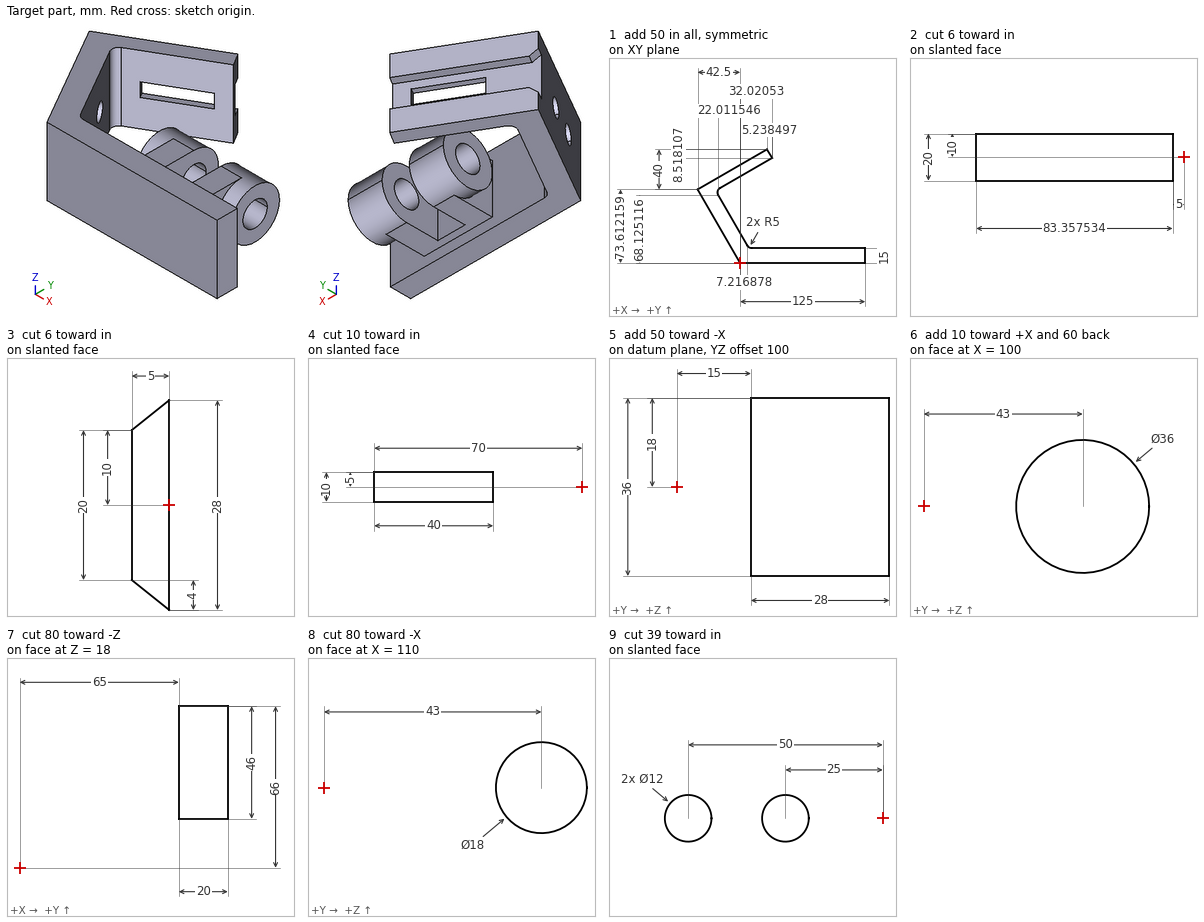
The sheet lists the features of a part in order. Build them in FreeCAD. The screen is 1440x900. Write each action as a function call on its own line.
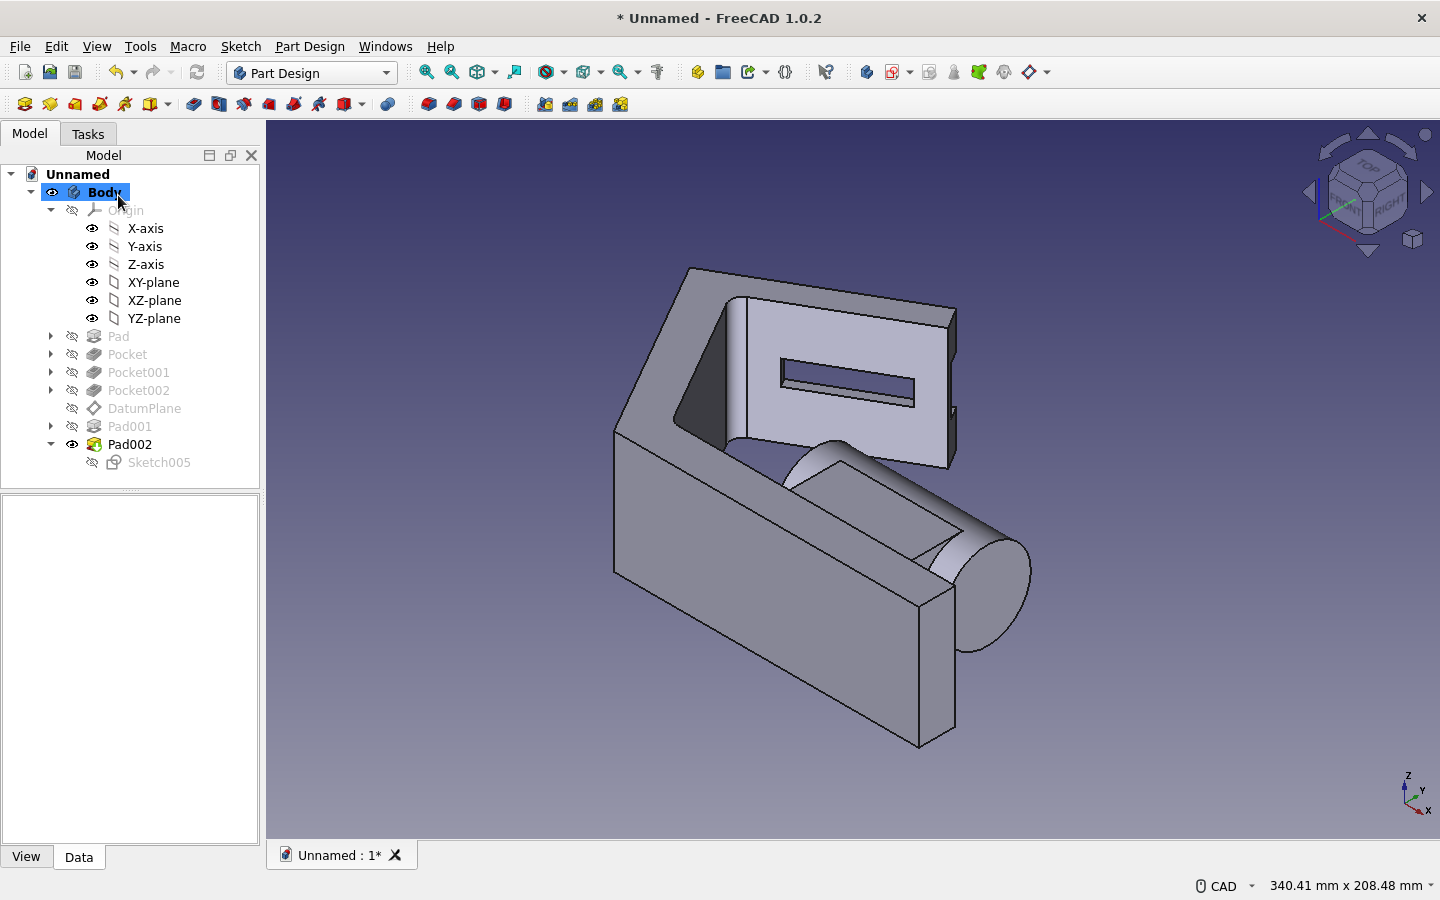
click(885, 525)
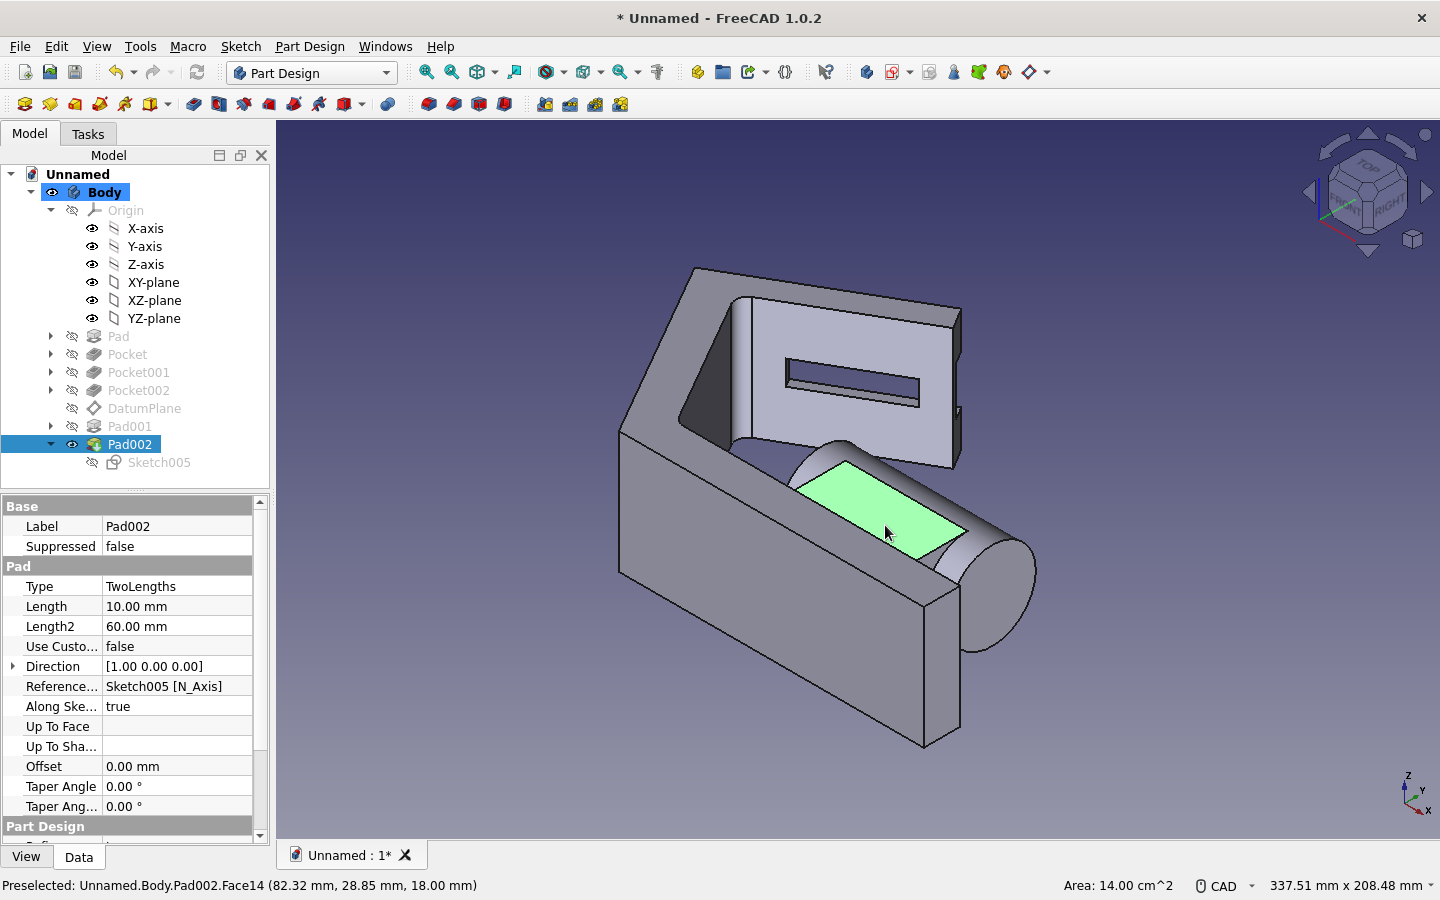
click(892, 72)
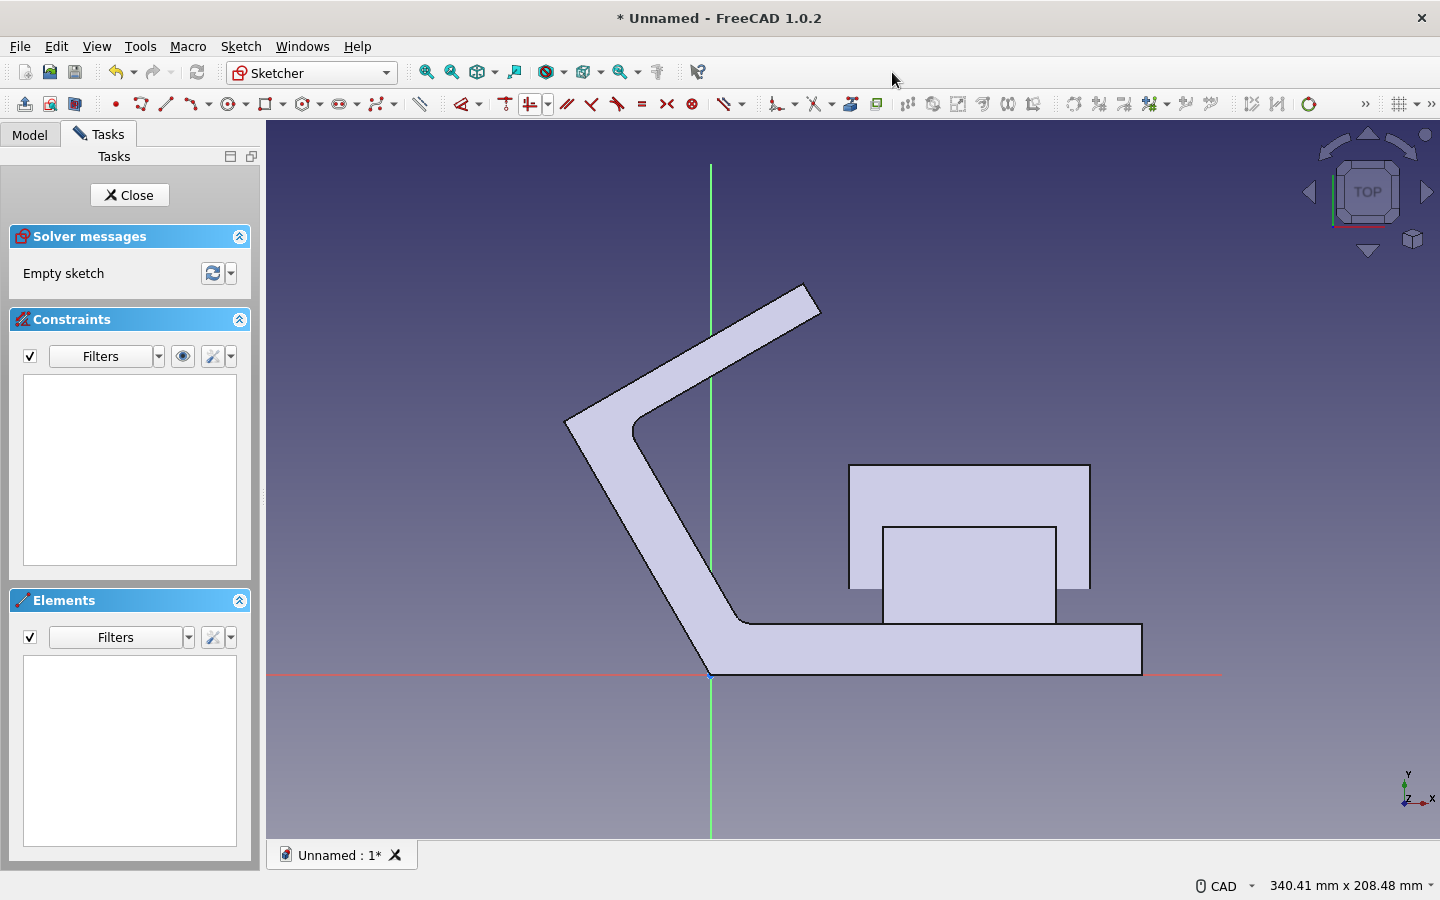
scroll(917, 629, up, 4)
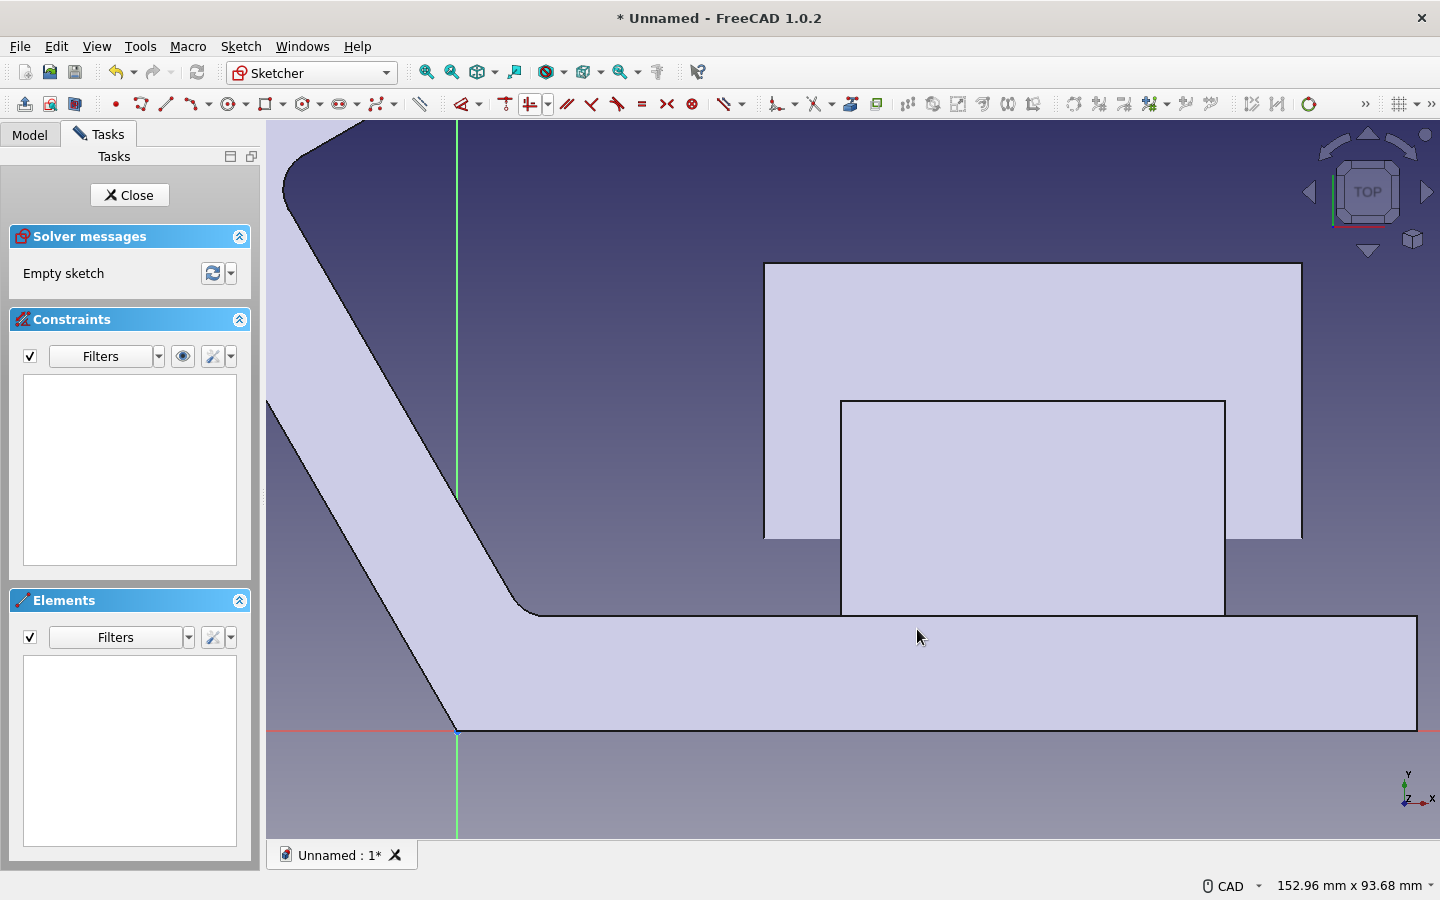
key(g)
key(r)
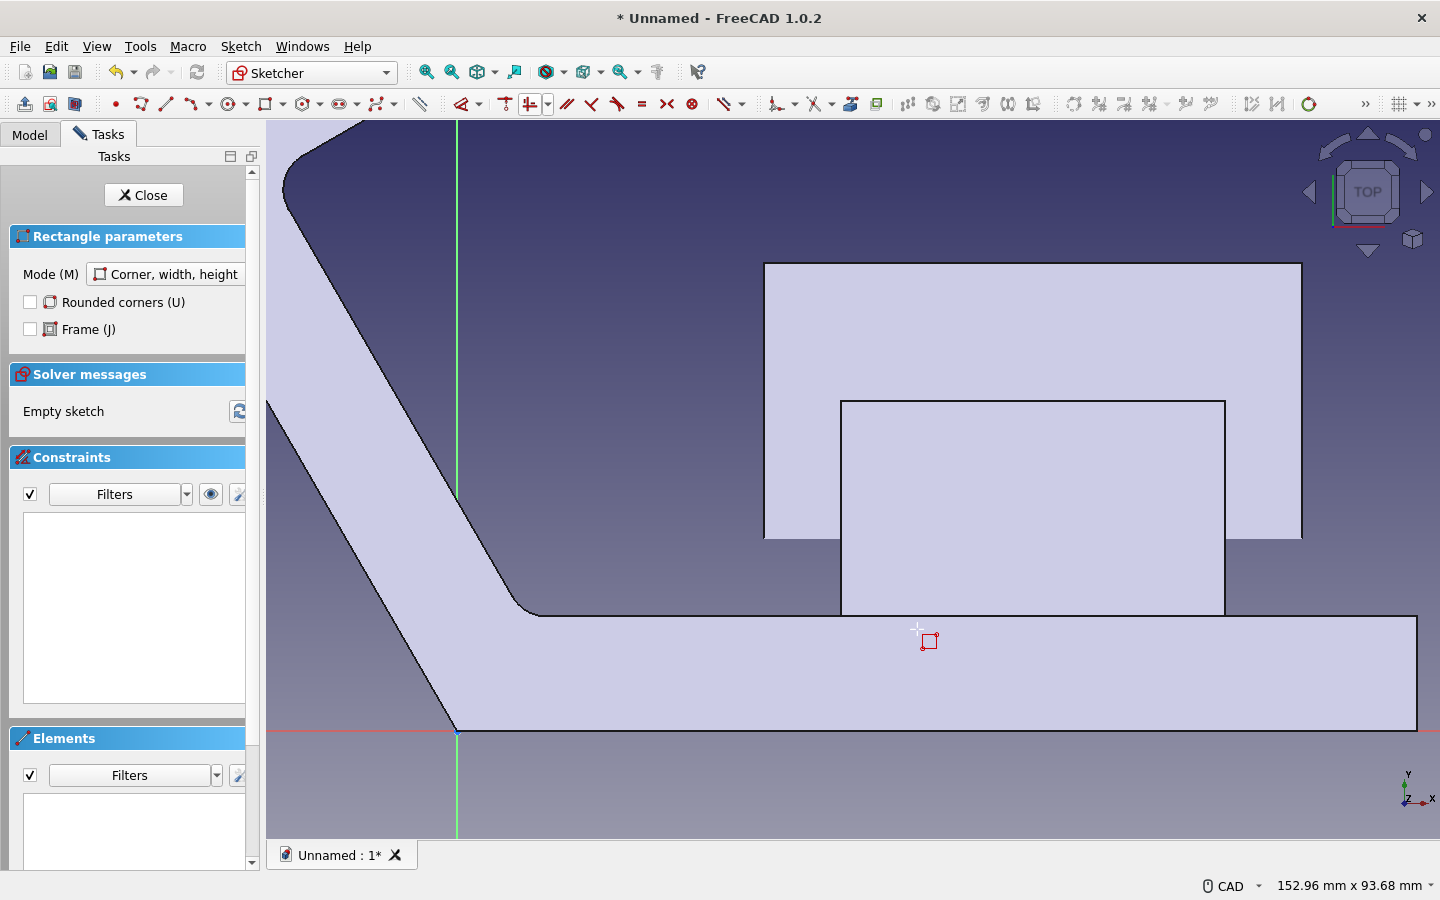
click(956, 225)
click(1110, 578)
key(Escape)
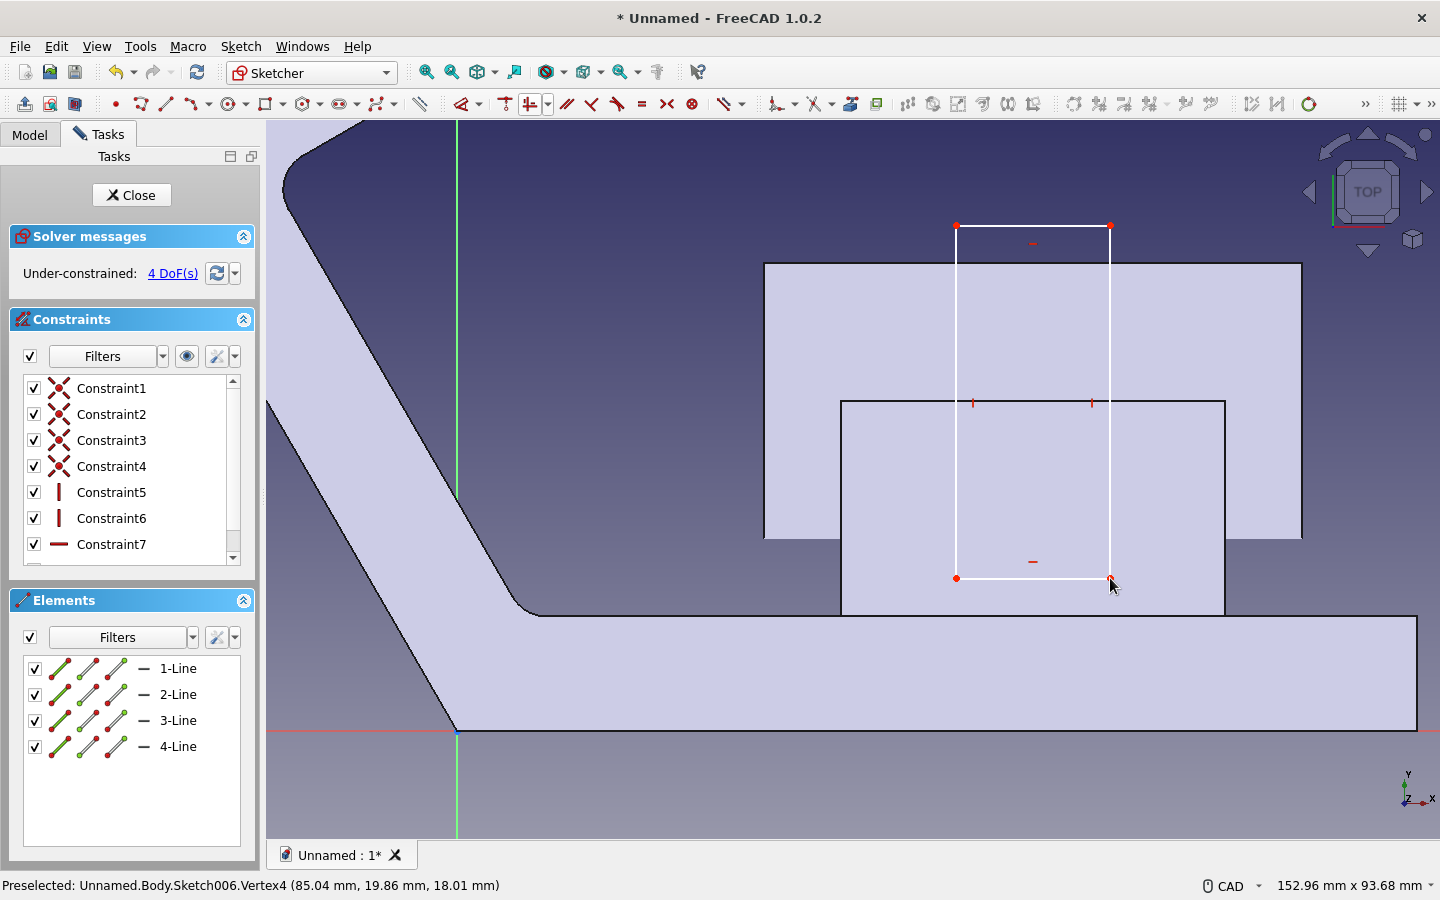
key(d)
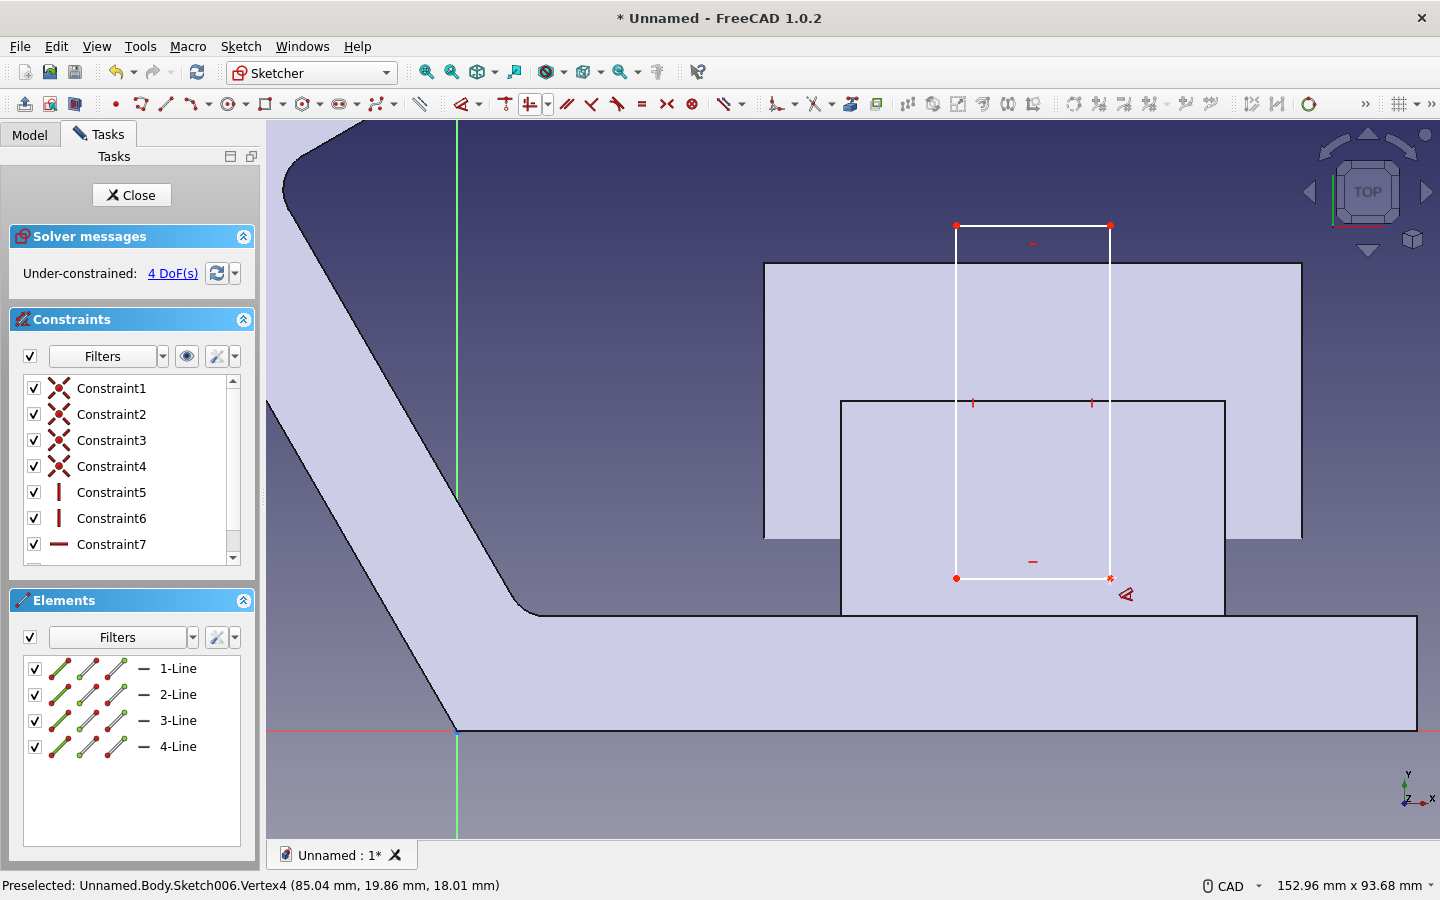
click(956, 332)
click(990, 402)